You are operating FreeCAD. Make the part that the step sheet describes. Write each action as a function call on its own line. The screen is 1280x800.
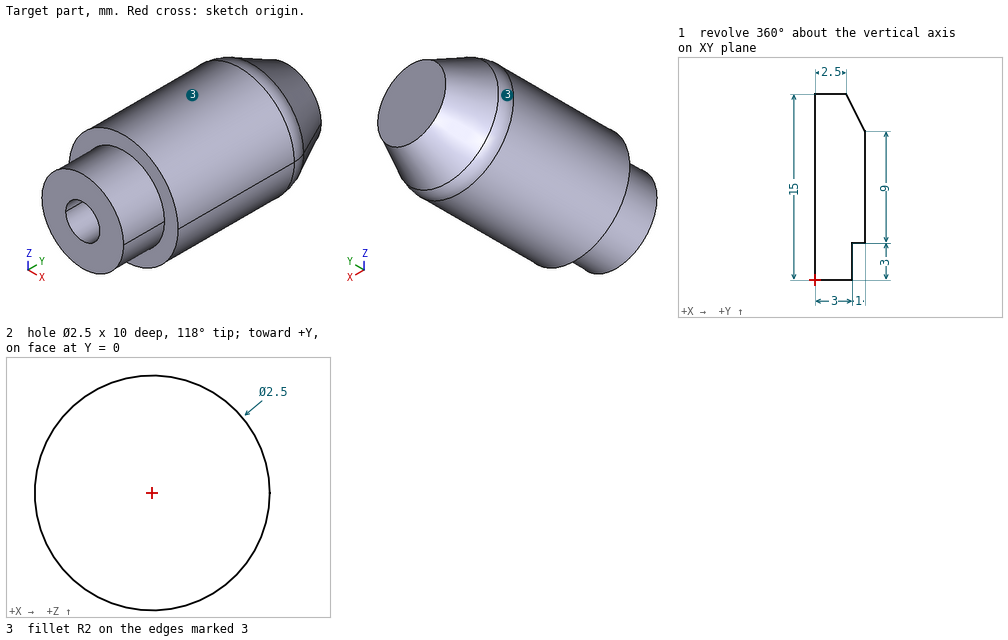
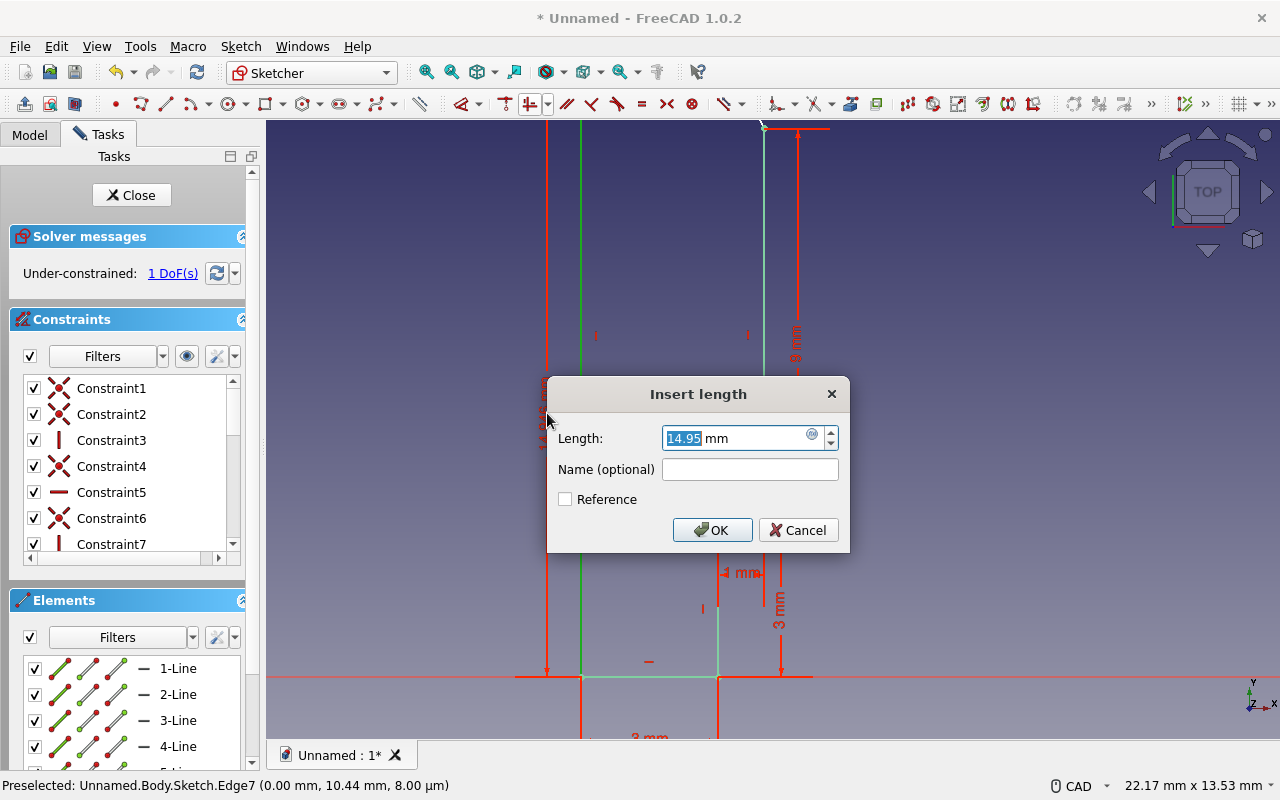
text(15)
key(Return)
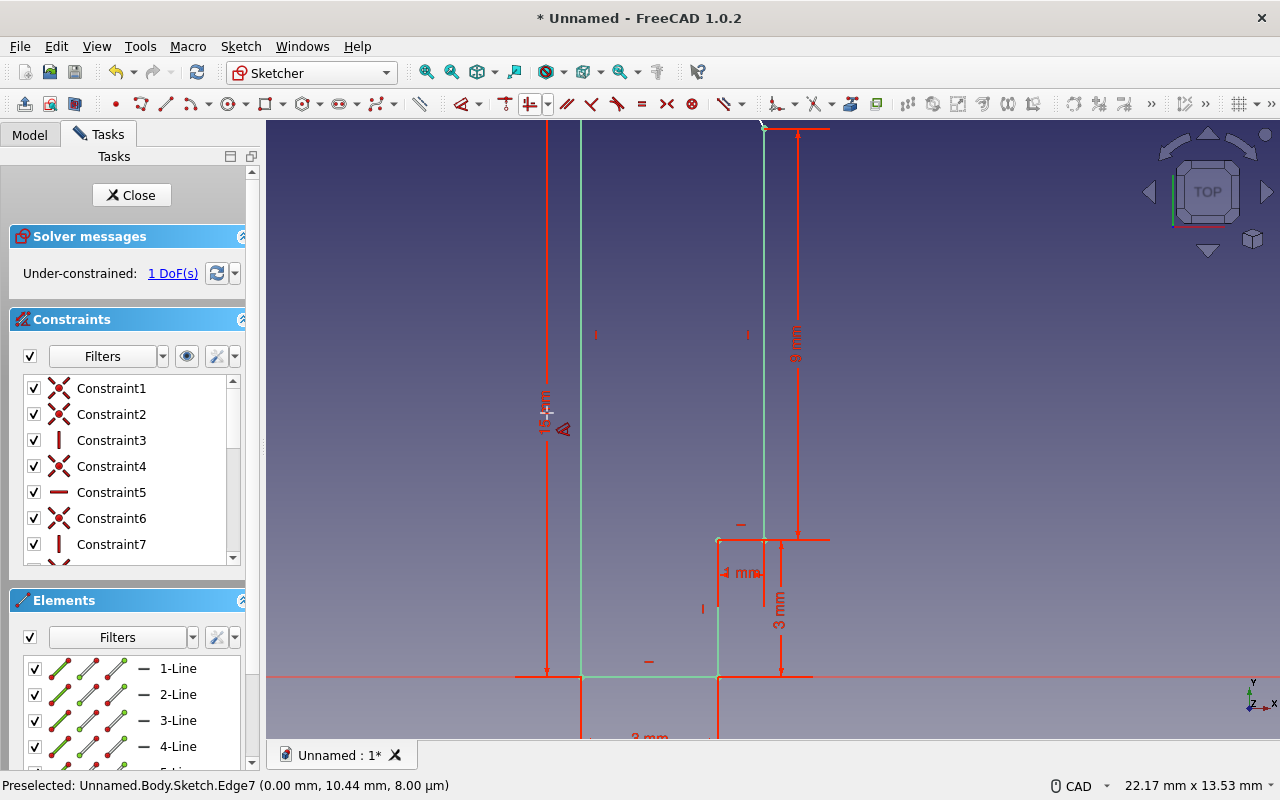
scroll(743, 545, down, 3)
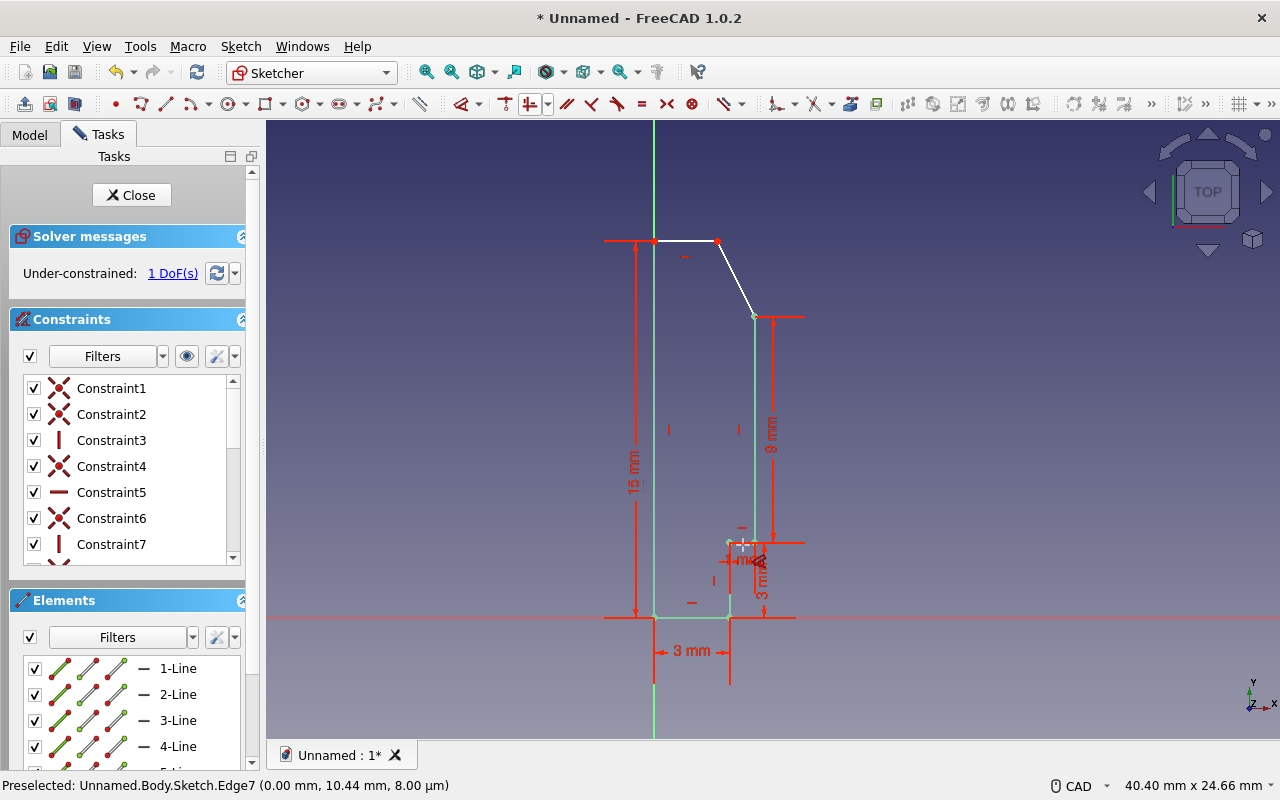
click(698, 241)
click(686, 207)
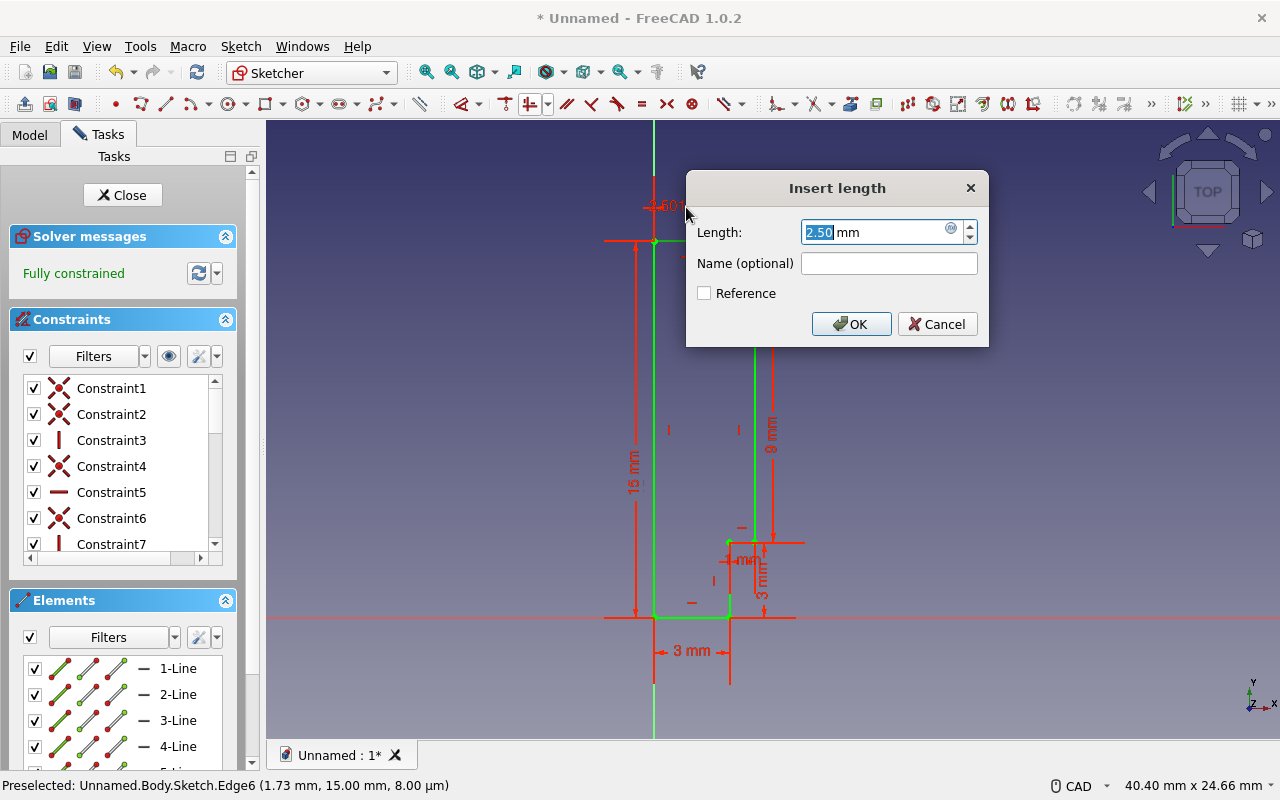
text(2.5)
key(Return)
key(Escape)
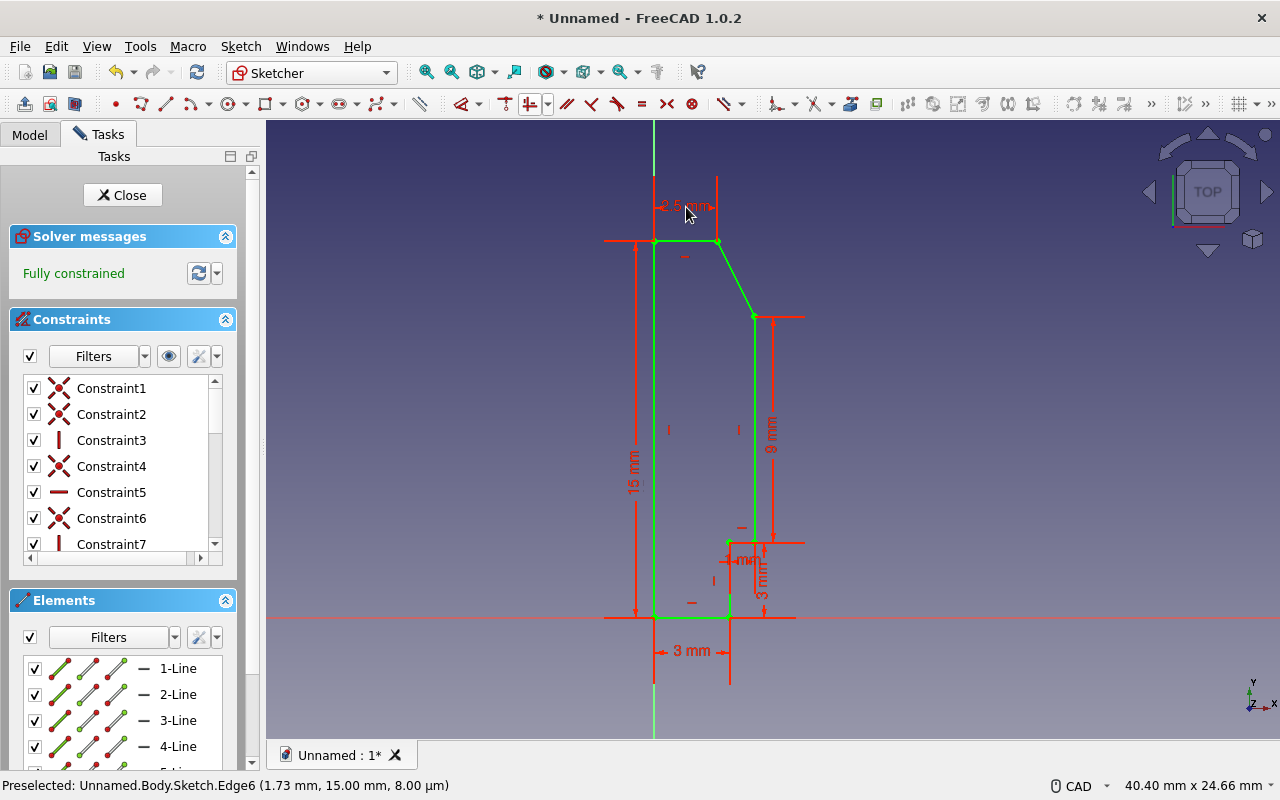
click(123, 195)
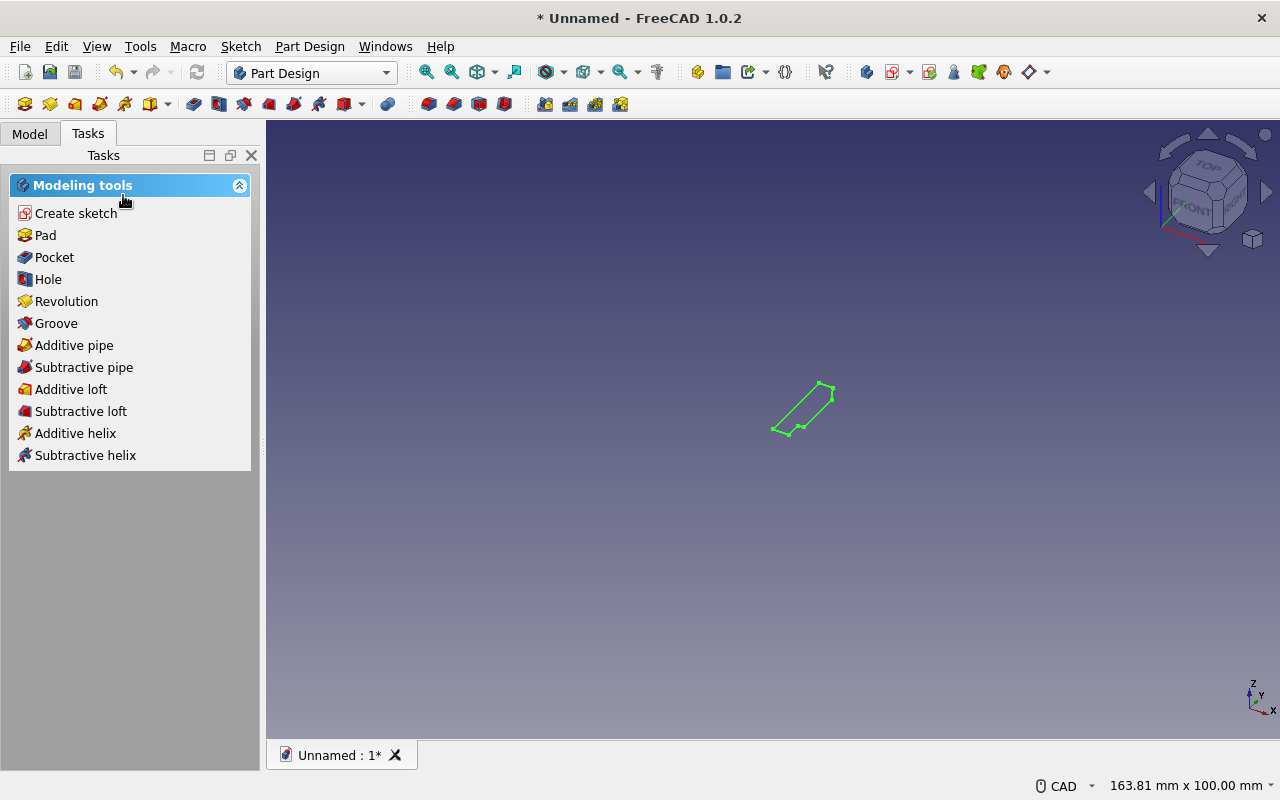
click(50, 104)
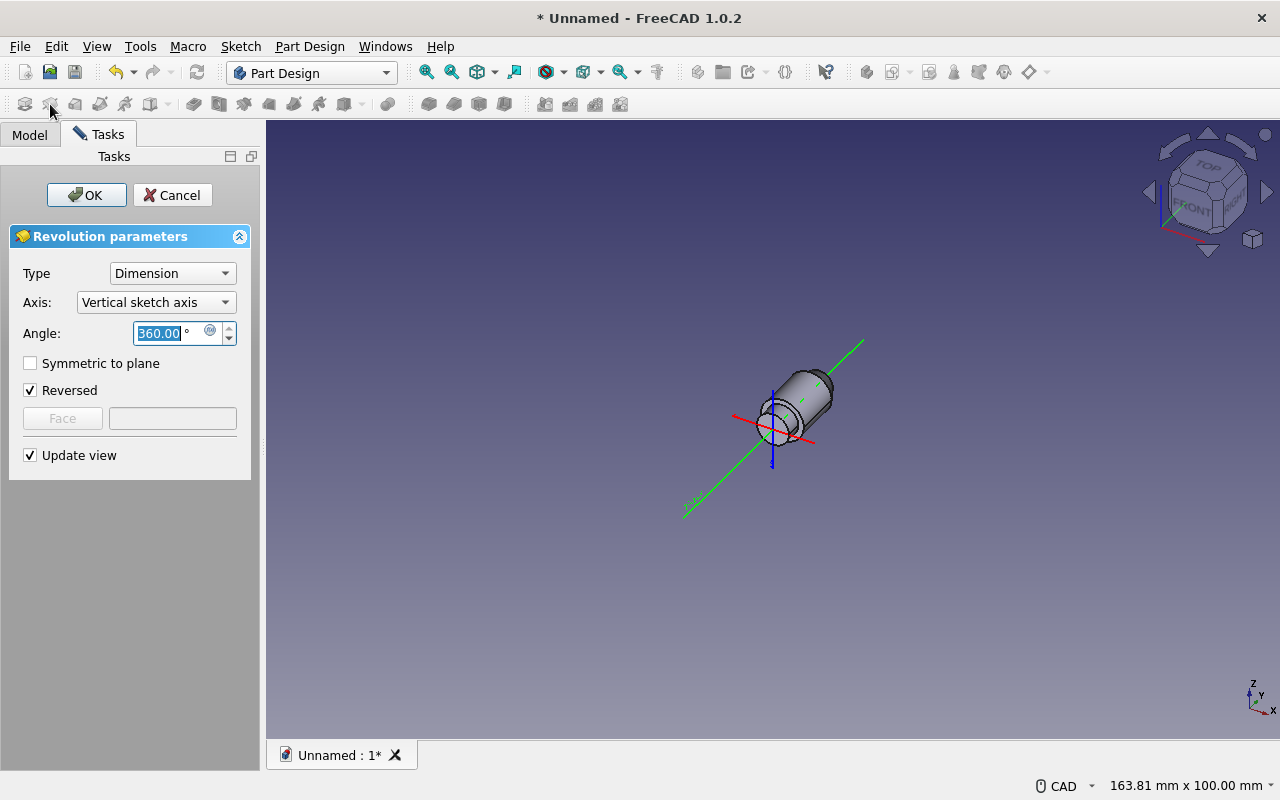
click(87, 195)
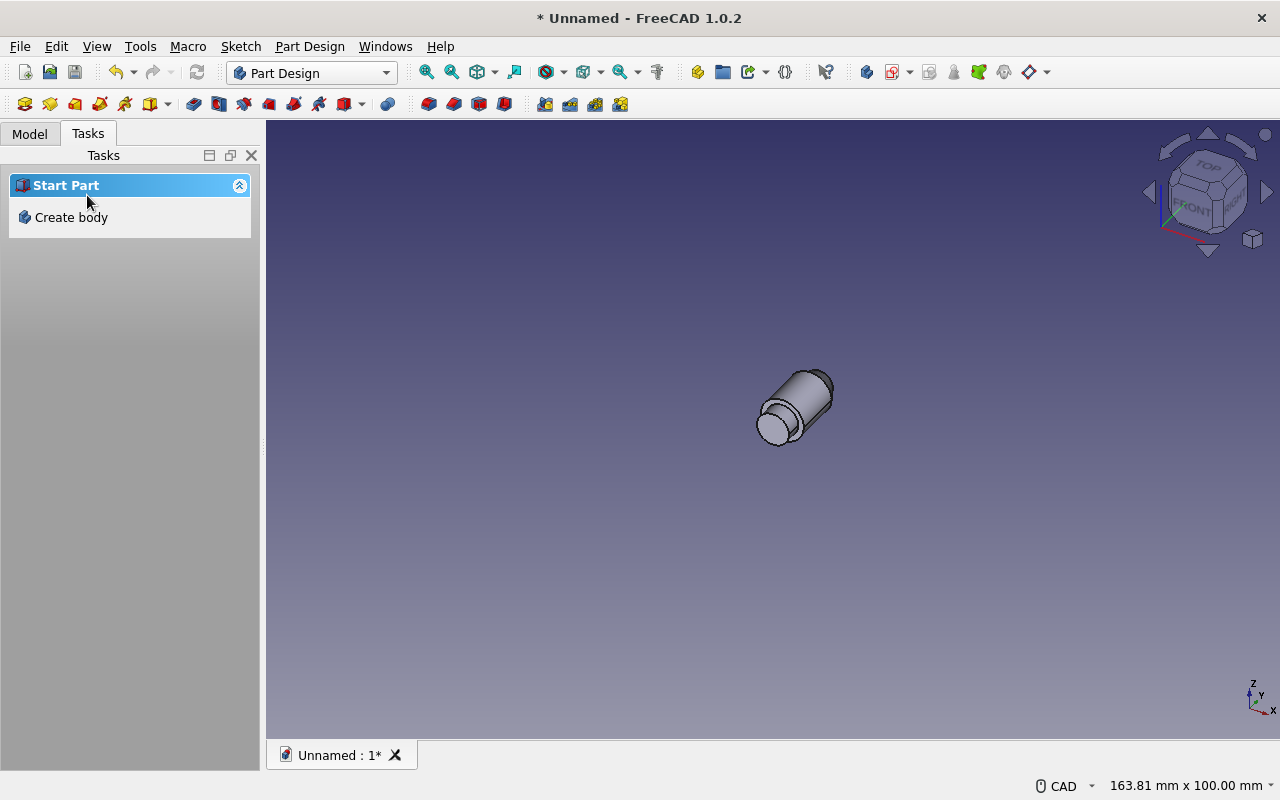
key(v)
key(f)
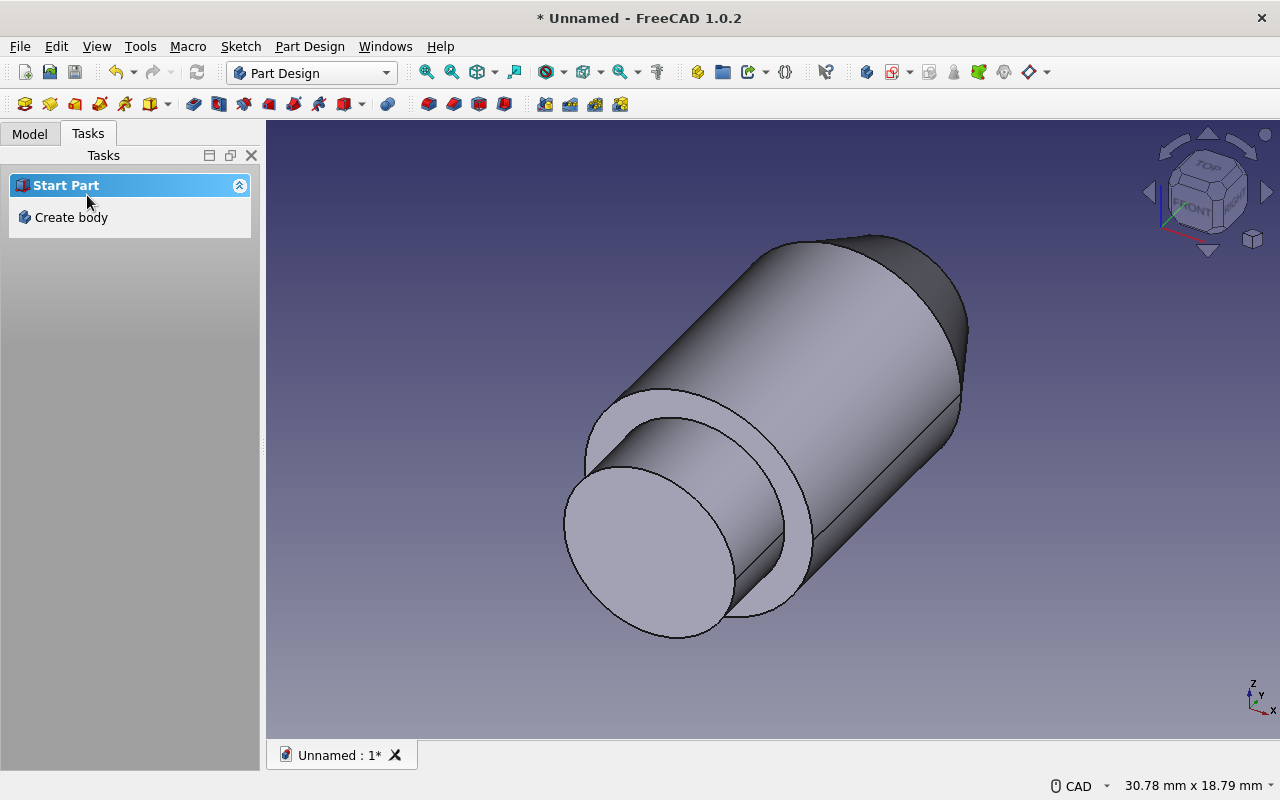
click(649, 551)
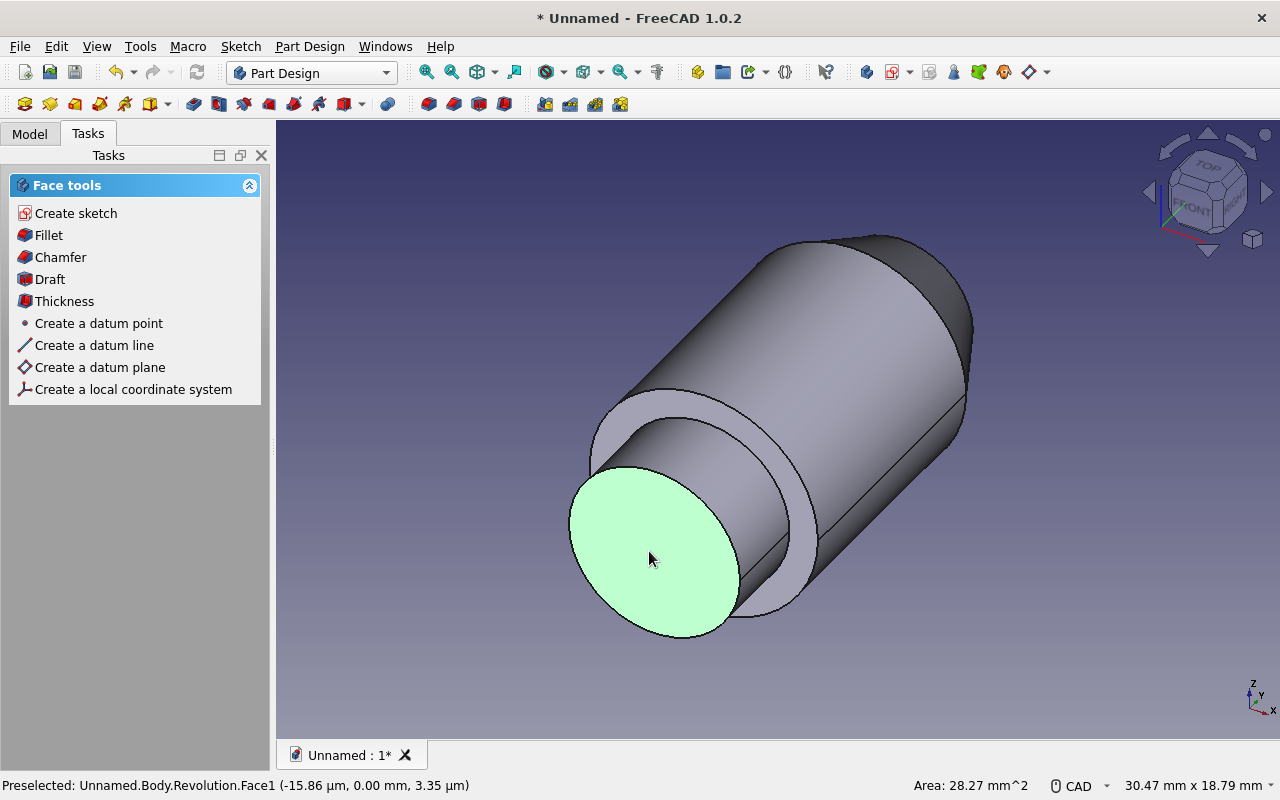
click(892, 72)